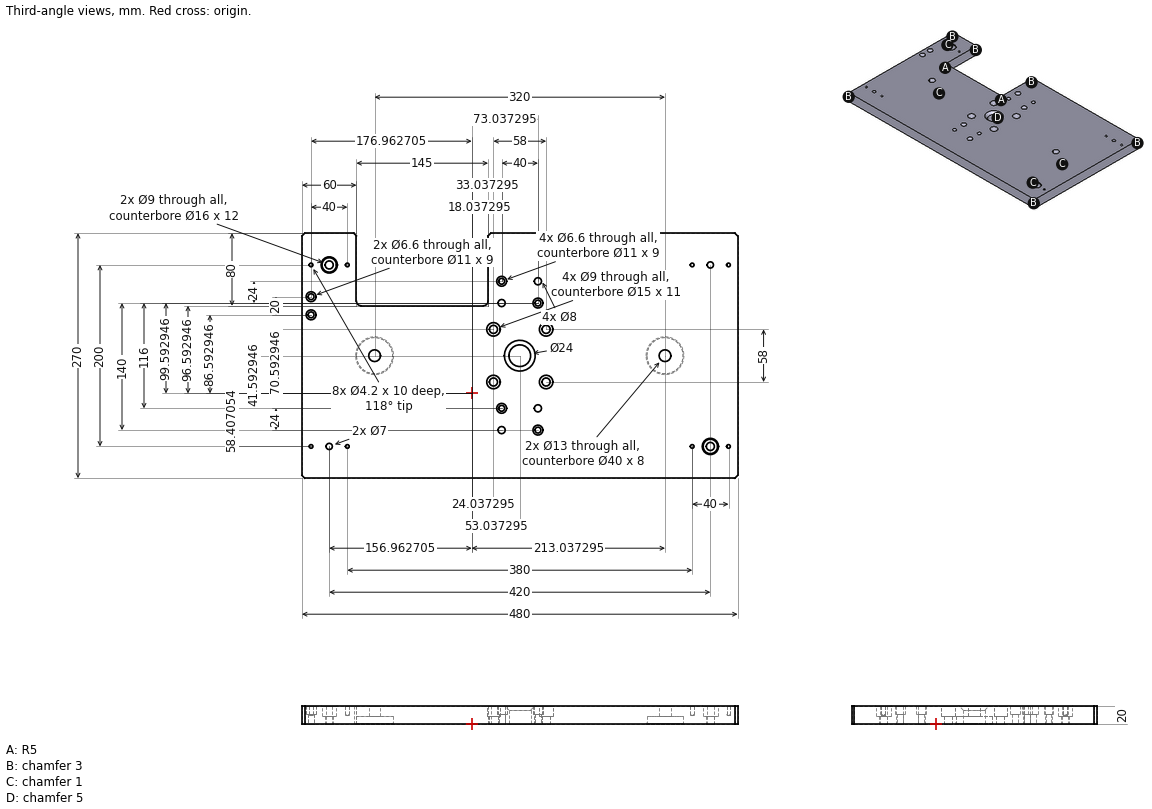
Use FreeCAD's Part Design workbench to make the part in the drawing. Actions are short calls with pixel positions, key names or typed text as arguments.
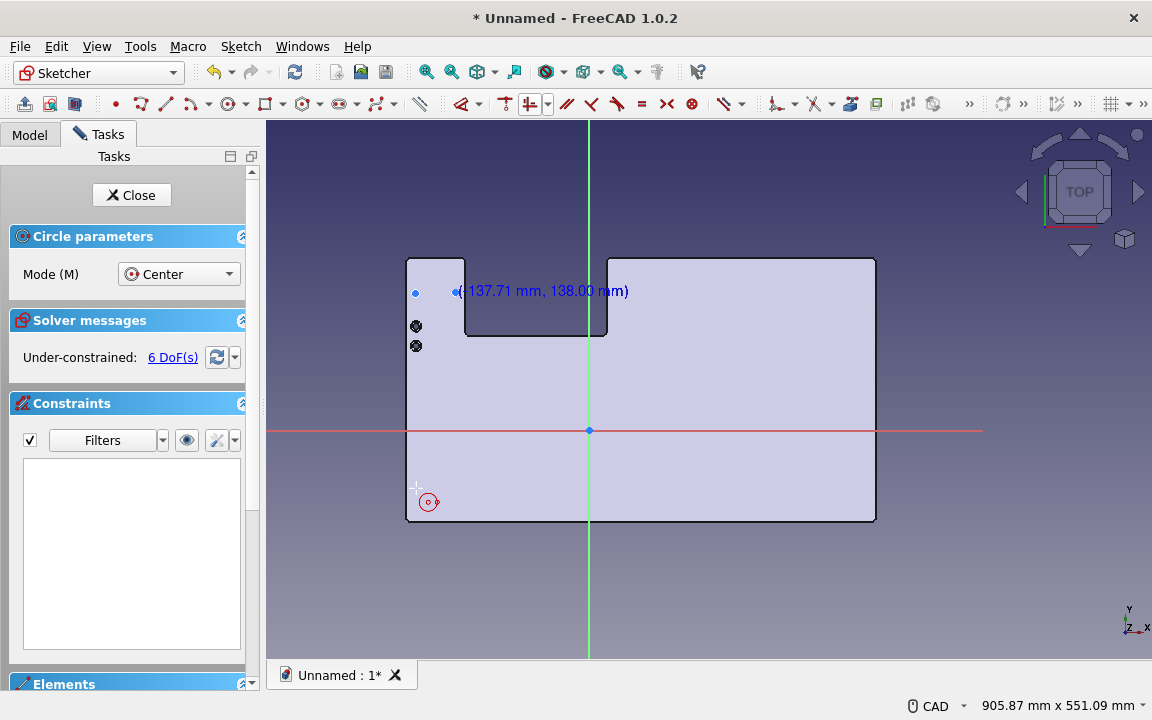
click(416, 488)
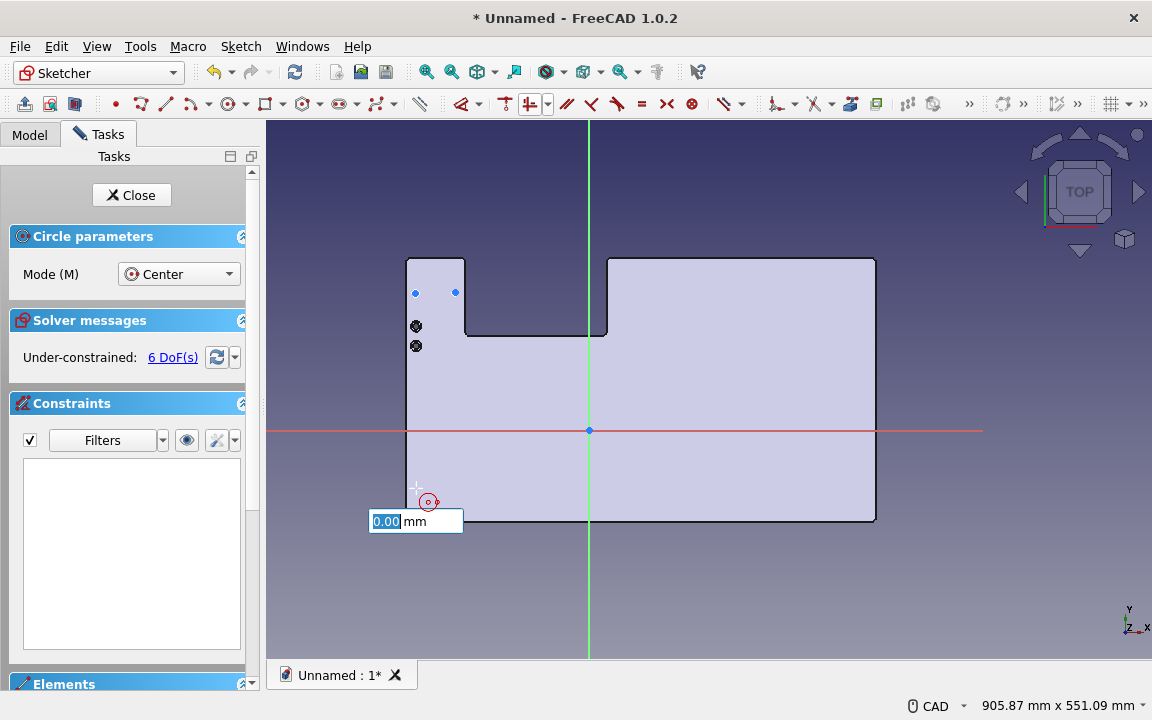
scroll(418, 486, up, 11)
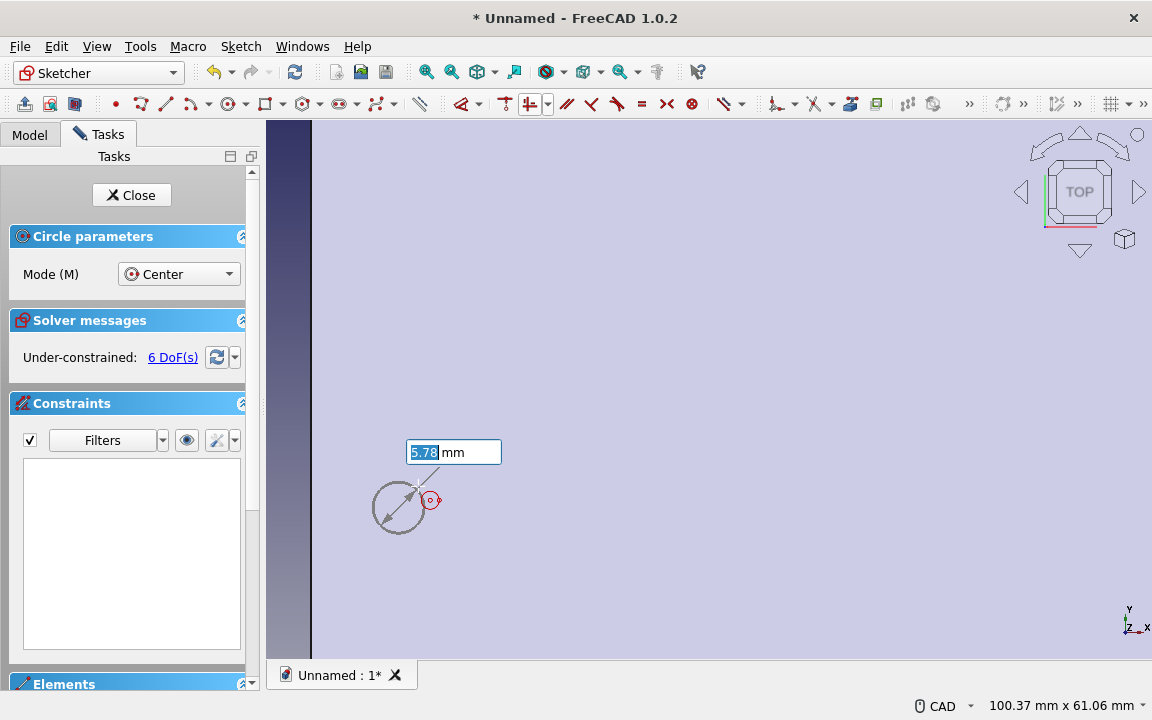
click(412, 483)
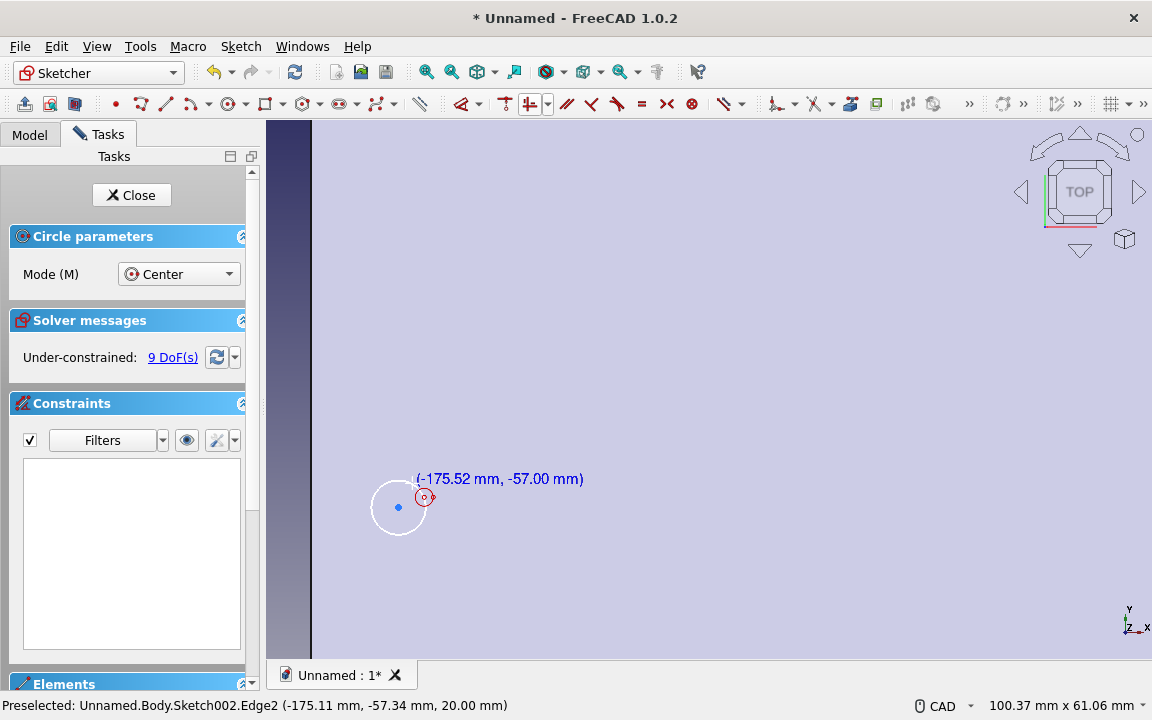
scroll(752, 496, up, 2)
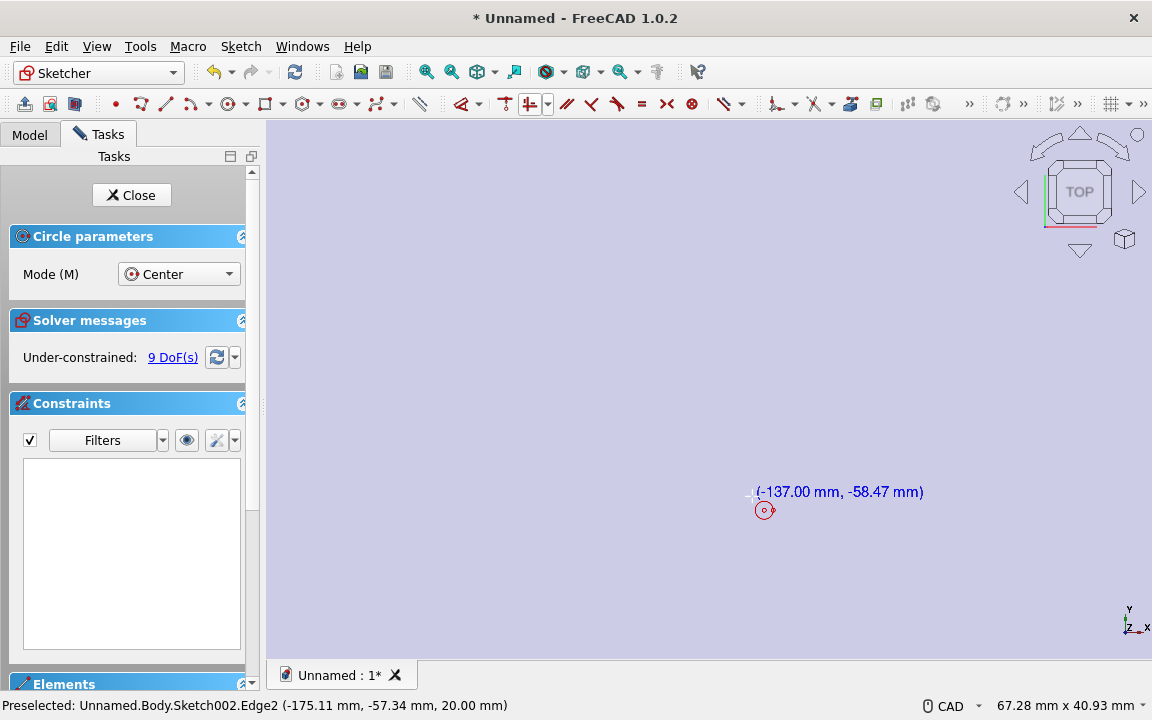
scroll(431, 487, down, 13)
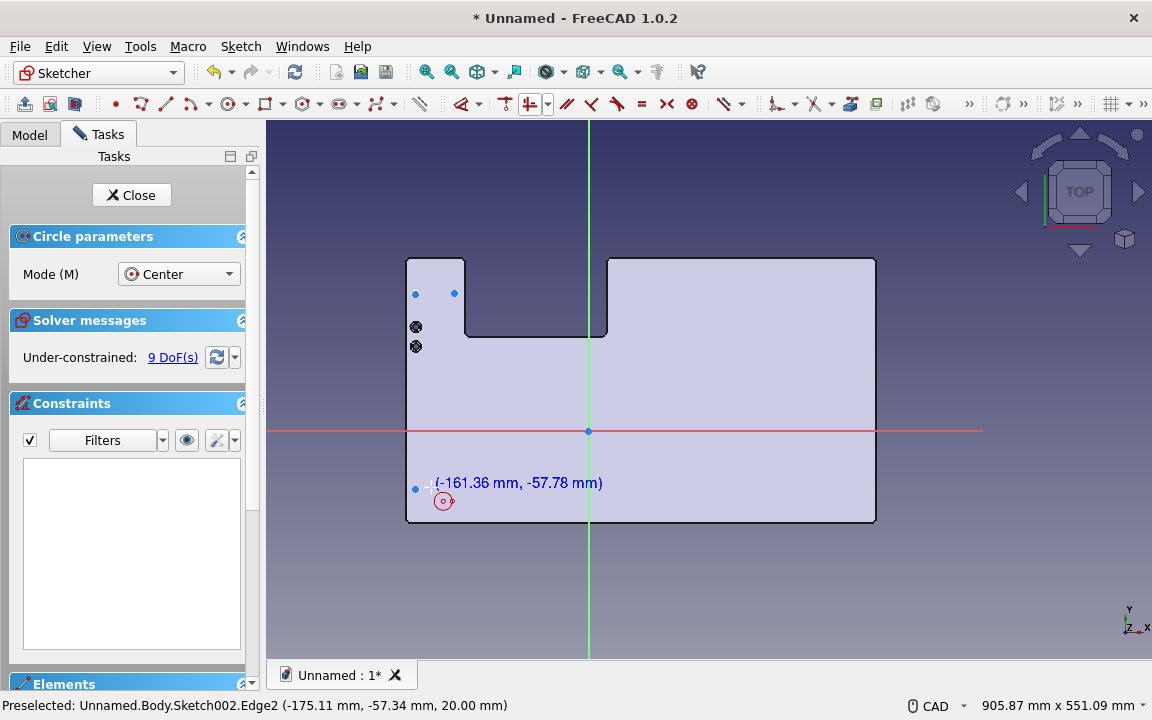
click(455, 488)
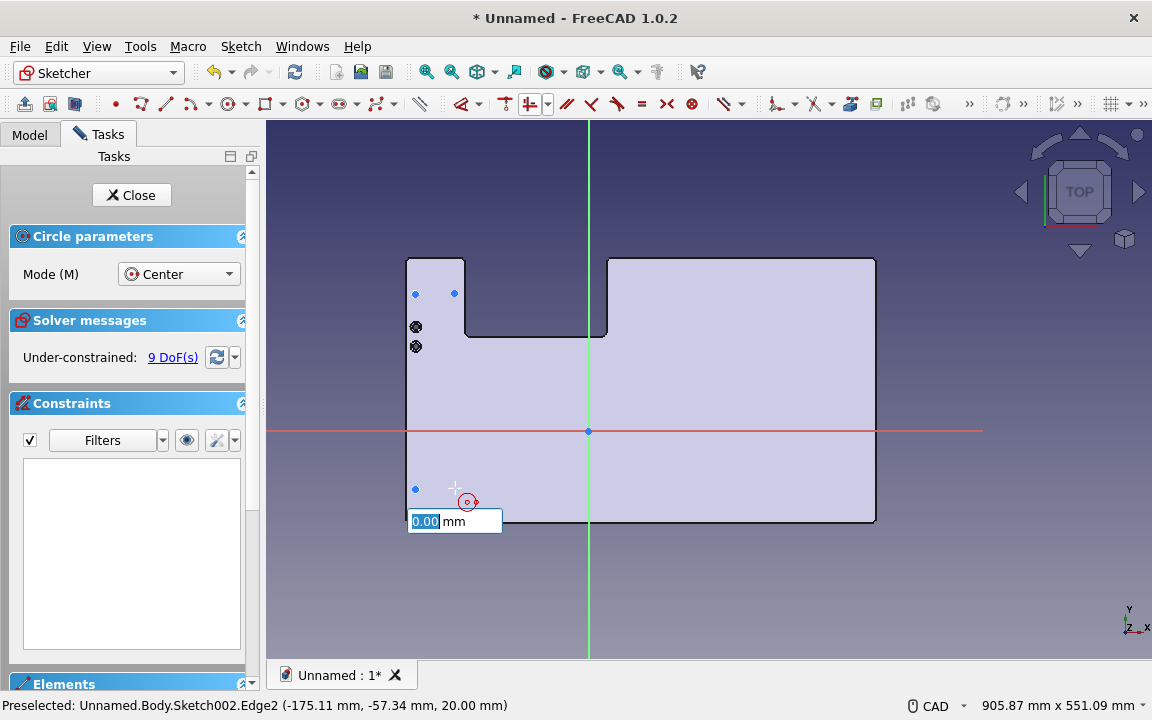
scroll(456, 487, up, 11)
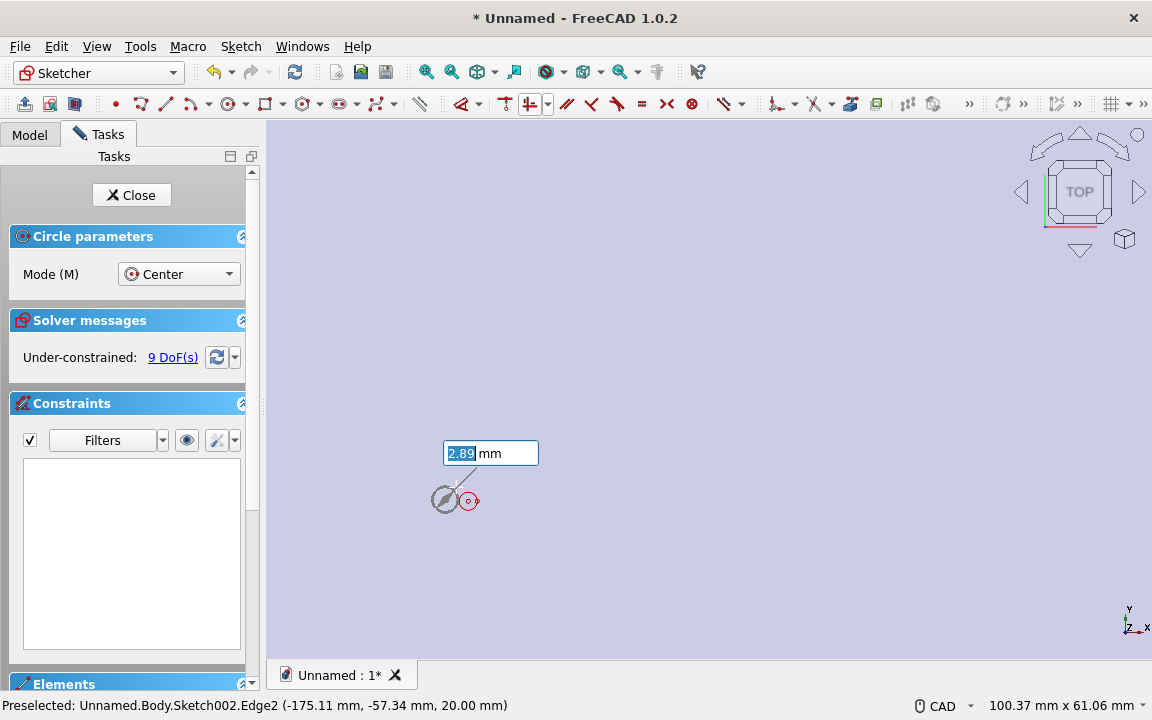
click(459, 480)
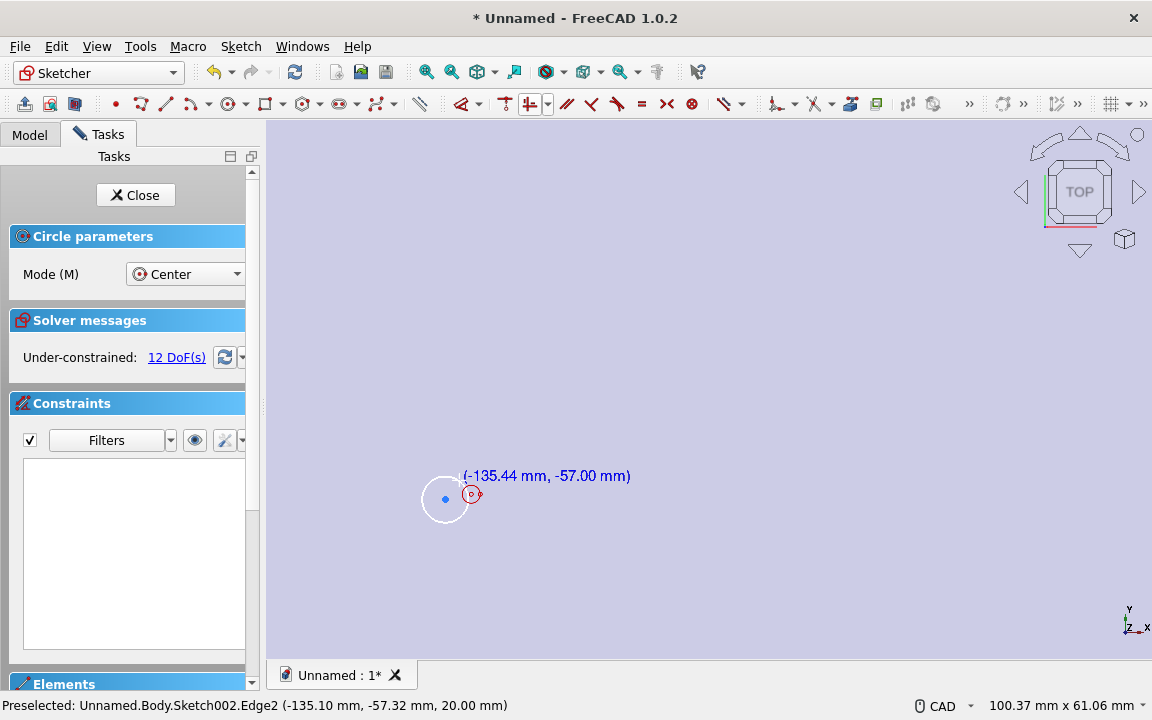
scroll(456, 487, down, 11)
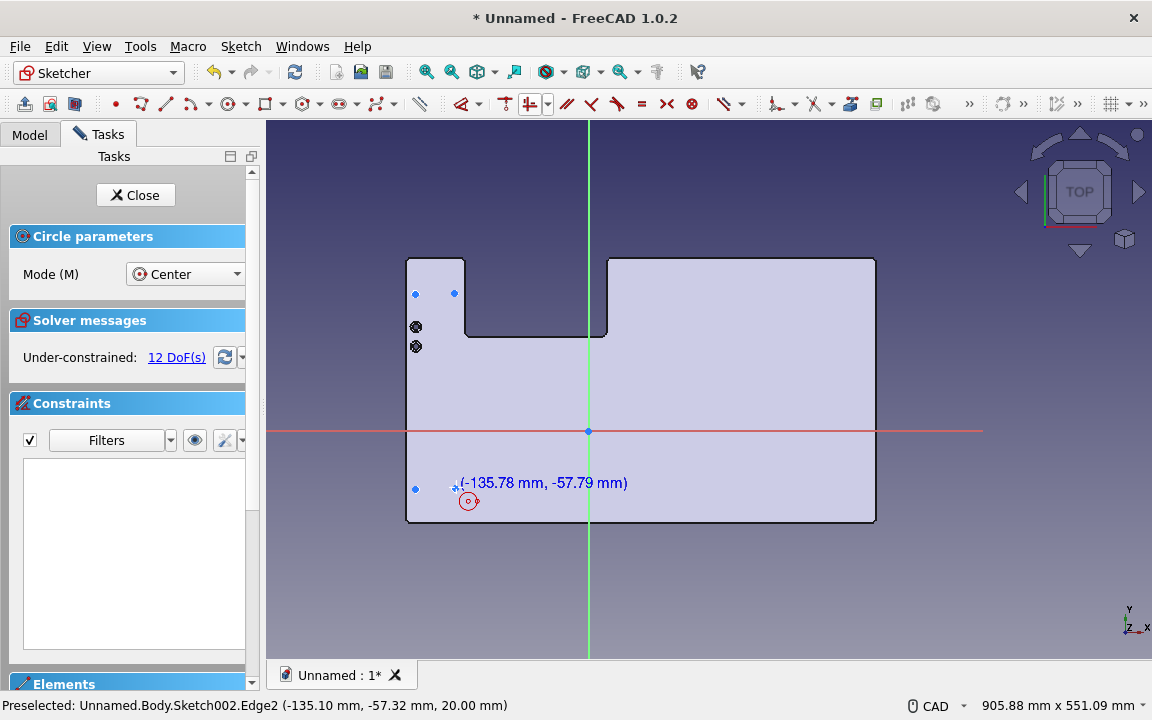
scroll(827, 488, up, 13)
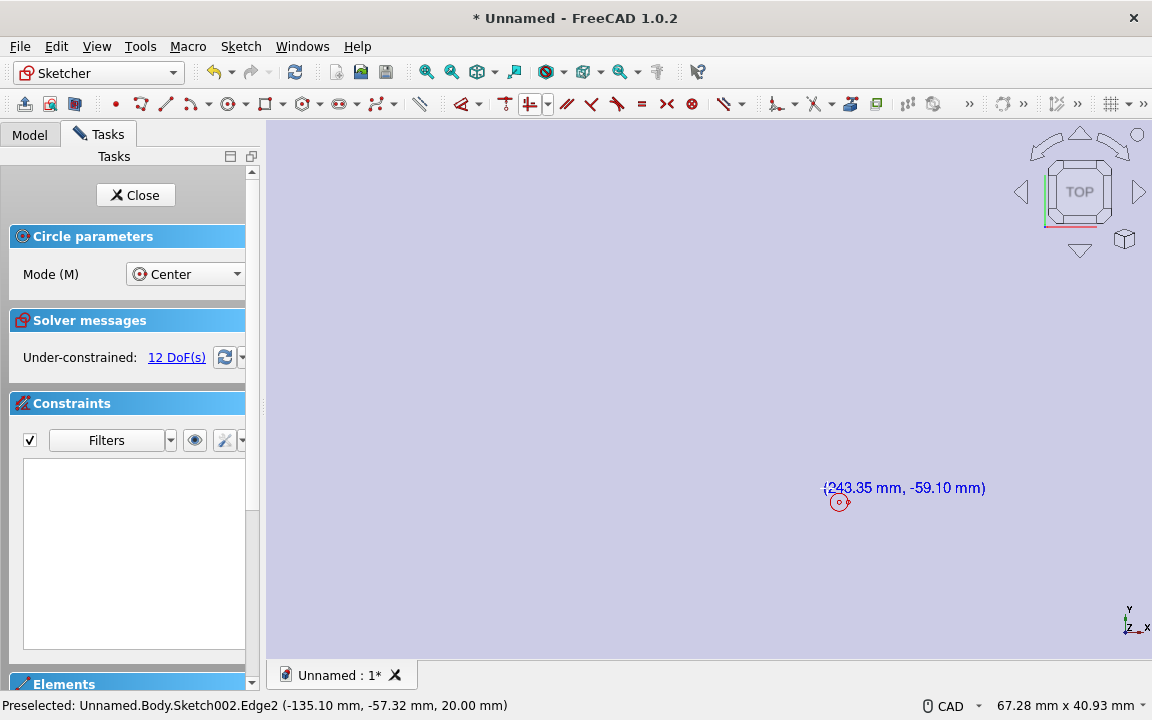
scroll(827, 488, down, 13)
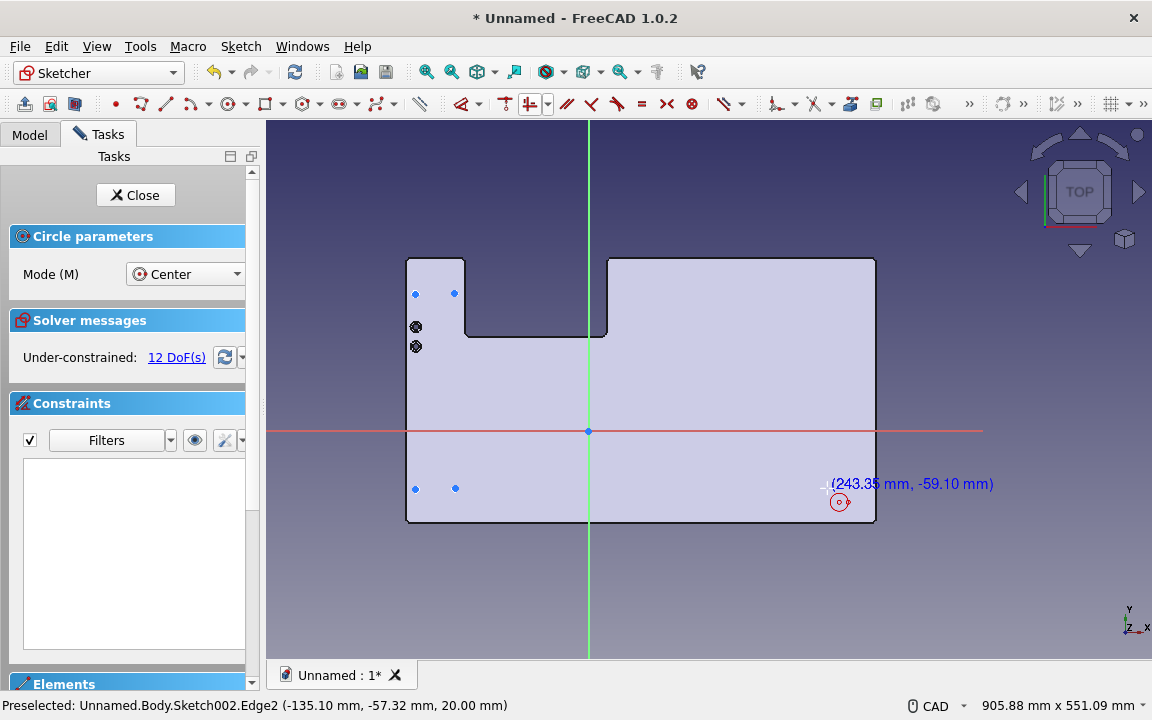
click(827, 488)